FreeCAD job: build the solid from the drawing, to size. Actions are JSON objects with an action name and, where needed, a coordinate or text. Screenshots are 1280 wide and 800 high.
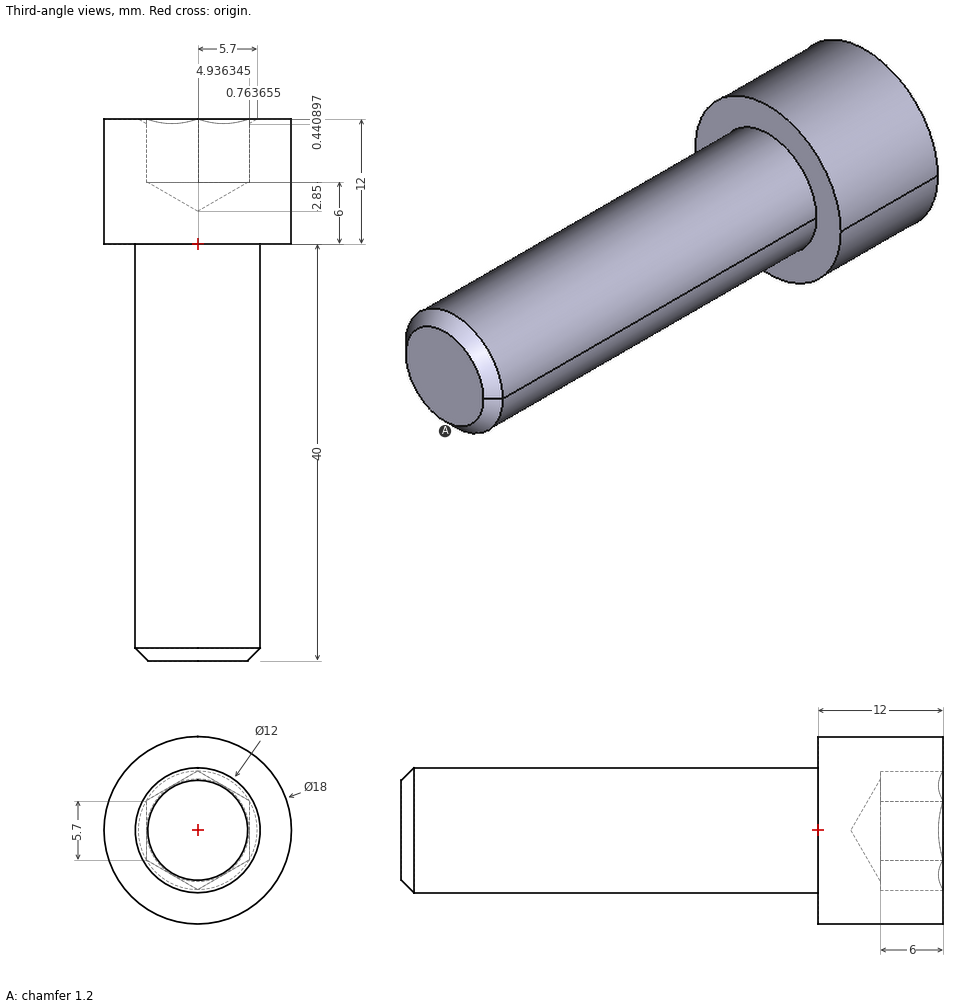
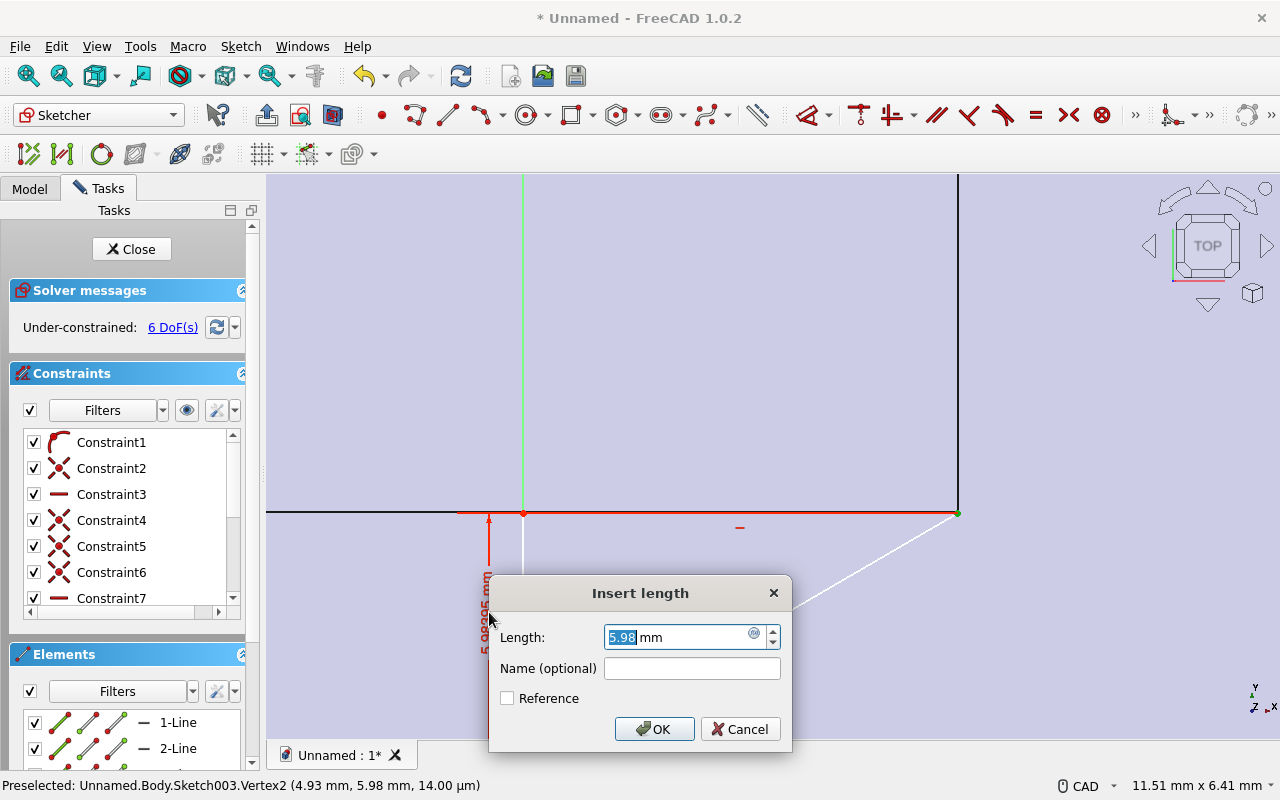
{"action": "type", "text": "6"}
{"action": "key", "text": "Return"}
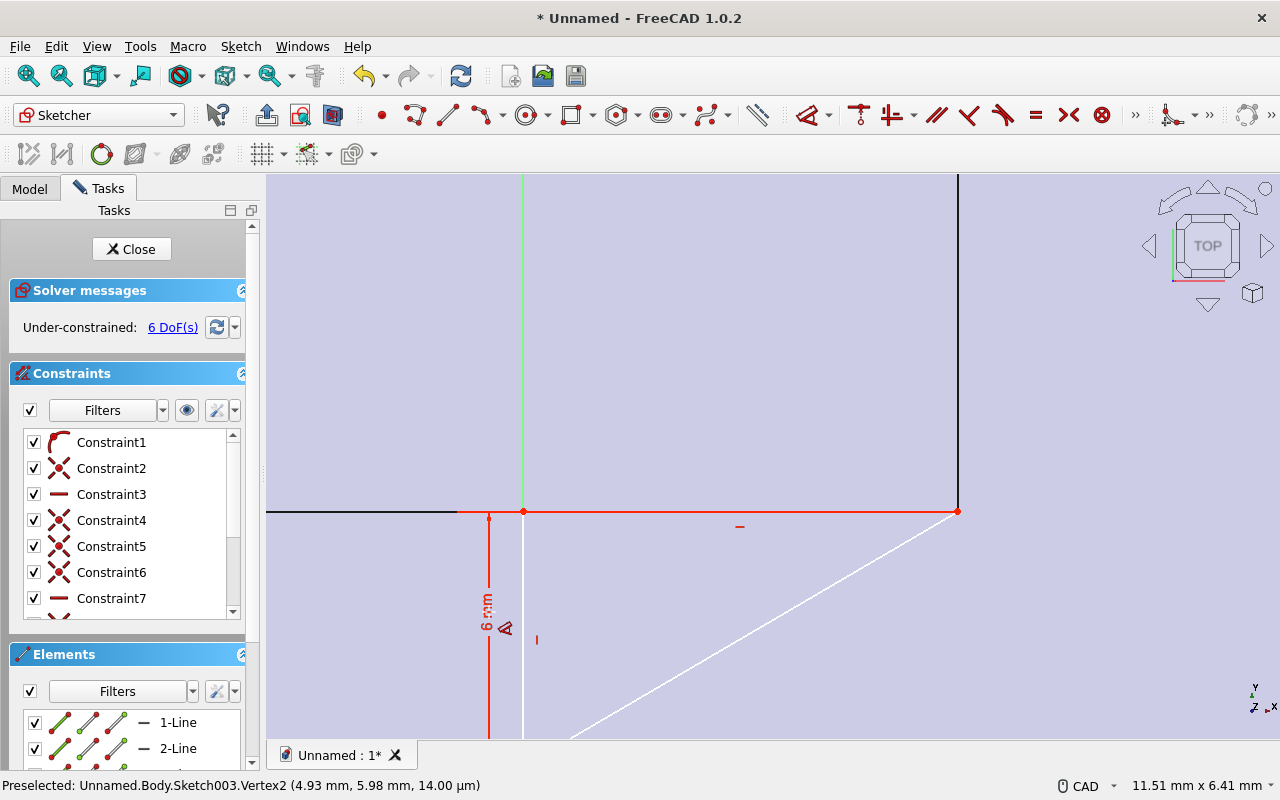
{"action": "scroll", "coordinate": [664, 424], "scroll_direction": "down", "scroll_amount": 5}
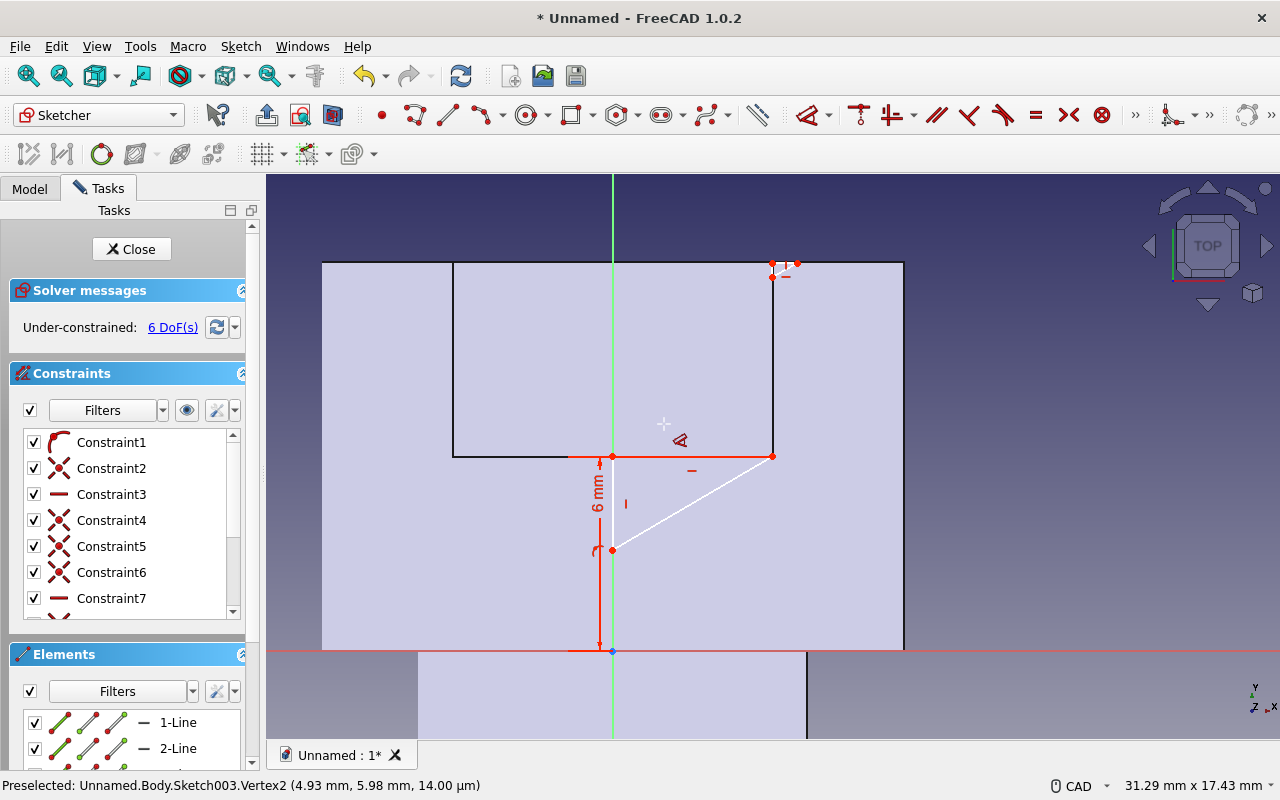
{"action": "left_click", "coordinate": [797, 263]}
{"action": "left_click", "coordinate": [579, 457]}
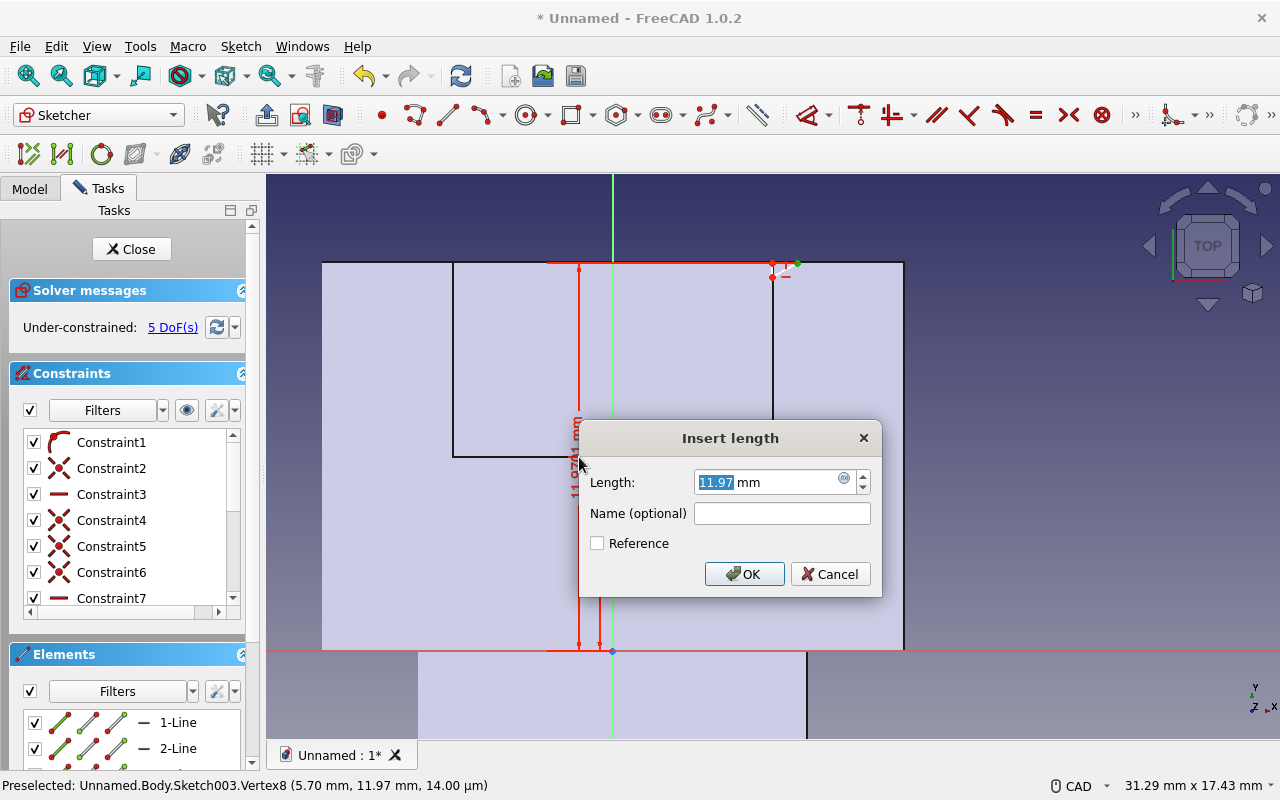
{"action": "type", "text": "12"}
{"action": "key", "text": "Return"}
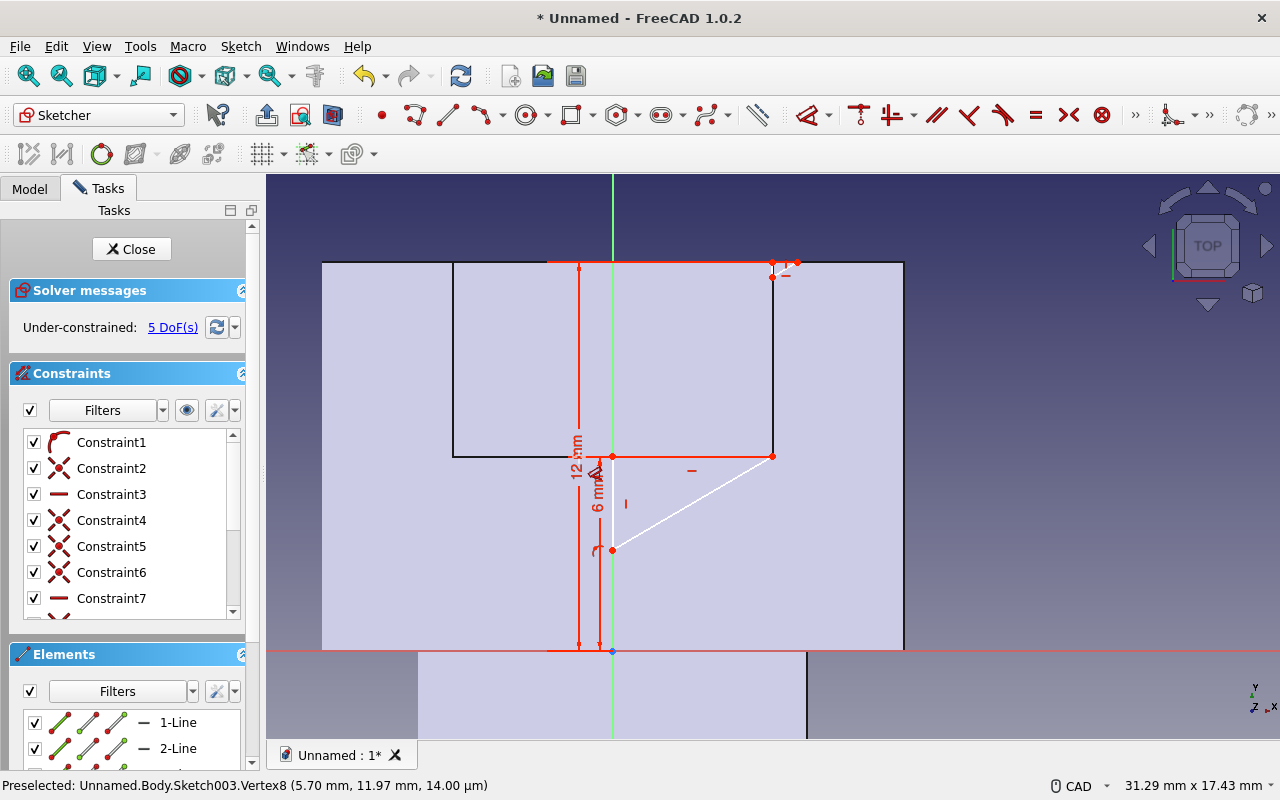
{"action": "left_click", "coordinate": [613, 485]}
{"action": "left_click", "coordinate": [579, 525]}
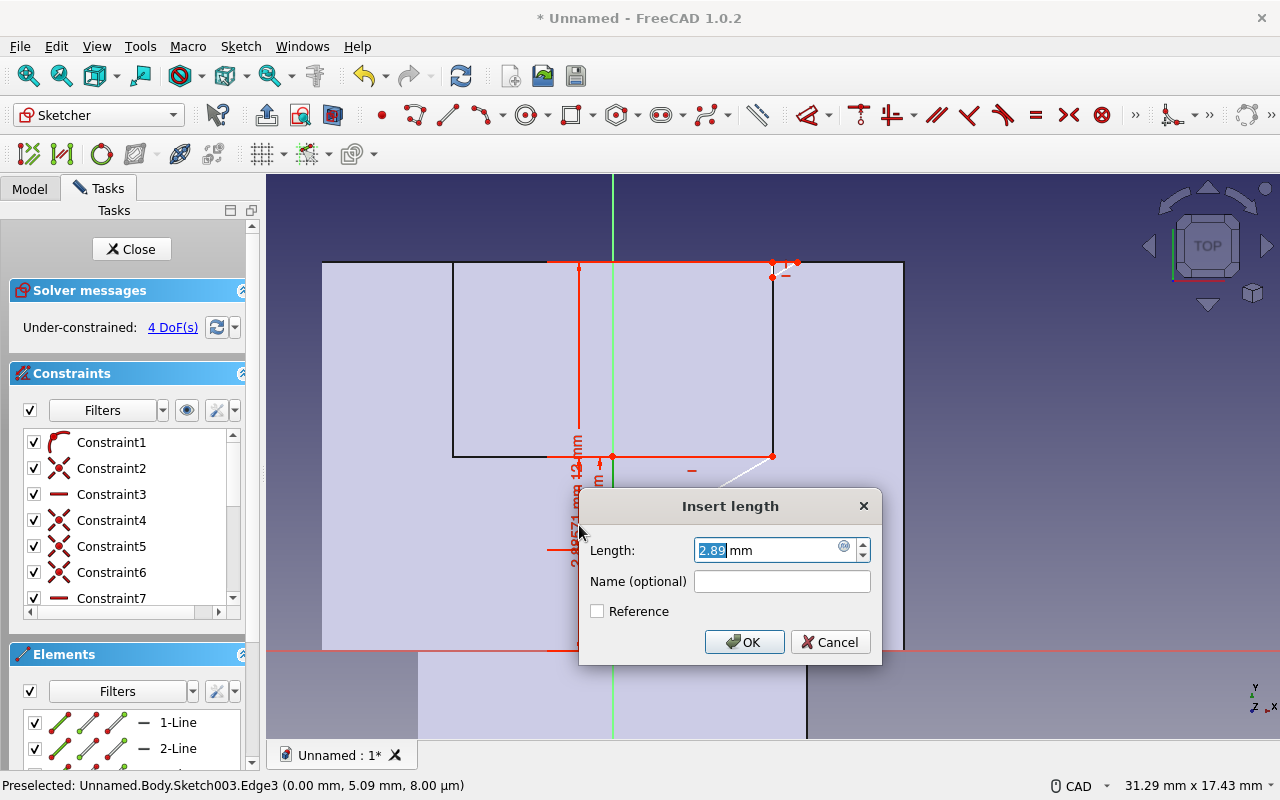
{"action": "type", "text": "2.85"}
{"action": "key", "text": "Return"}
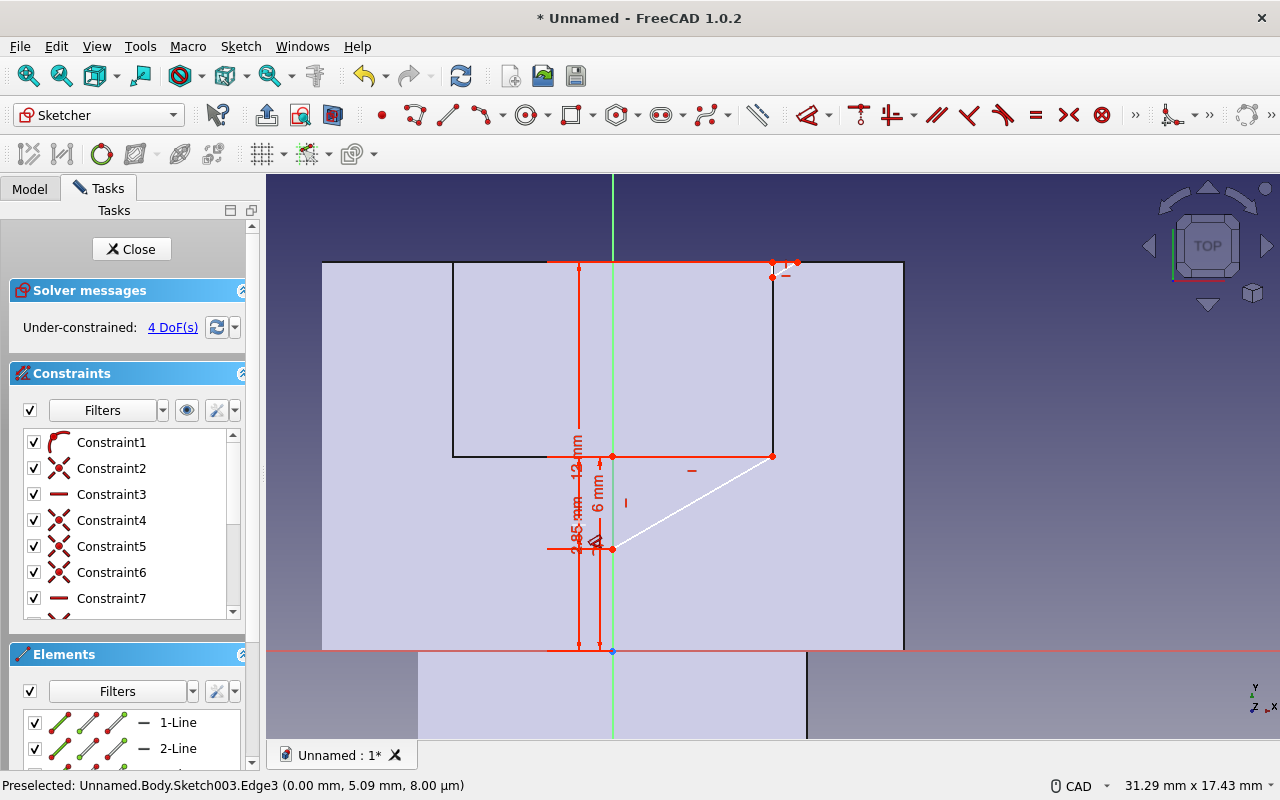
{"action": "left_click", "coordinate": [797, 262]}
{"action": "left_click", "coordinate": [705, 685]}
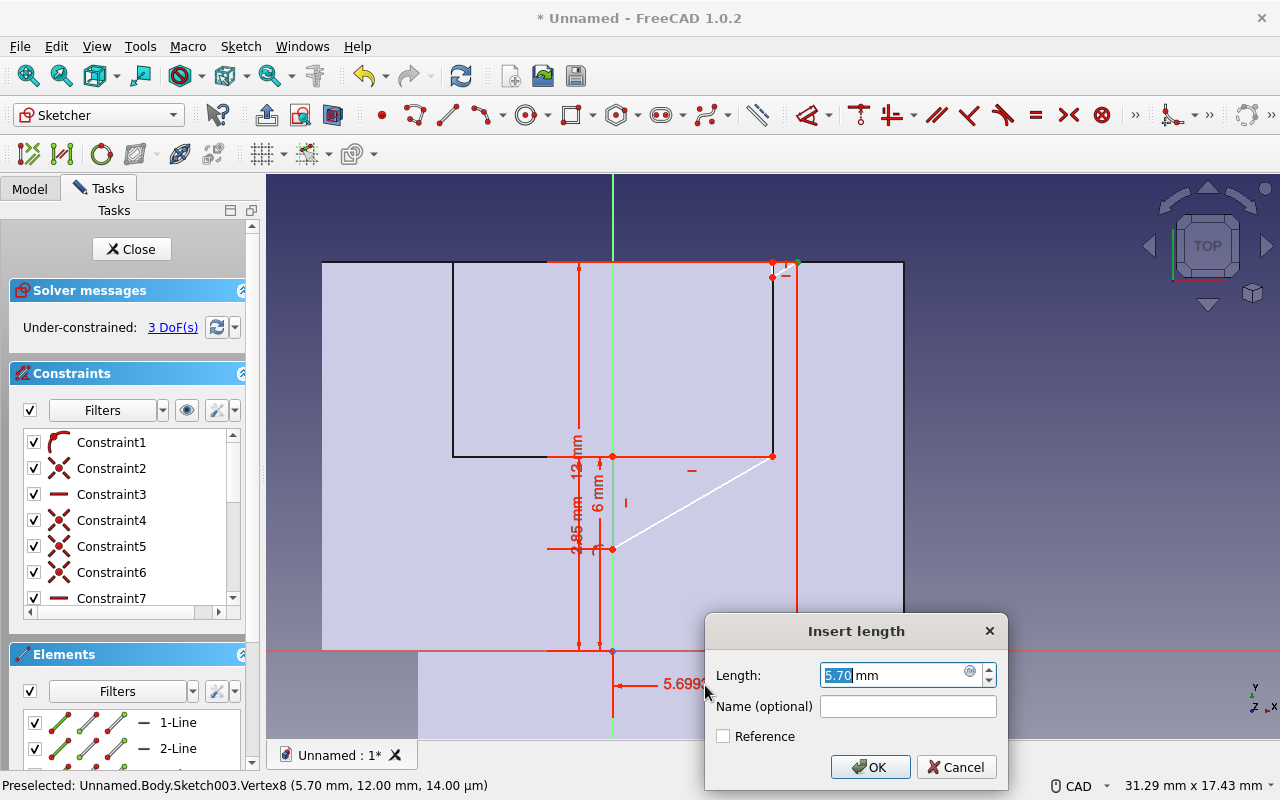
{"action": "type", "text": "5.7"}
{"action": "key", "text": "Return"}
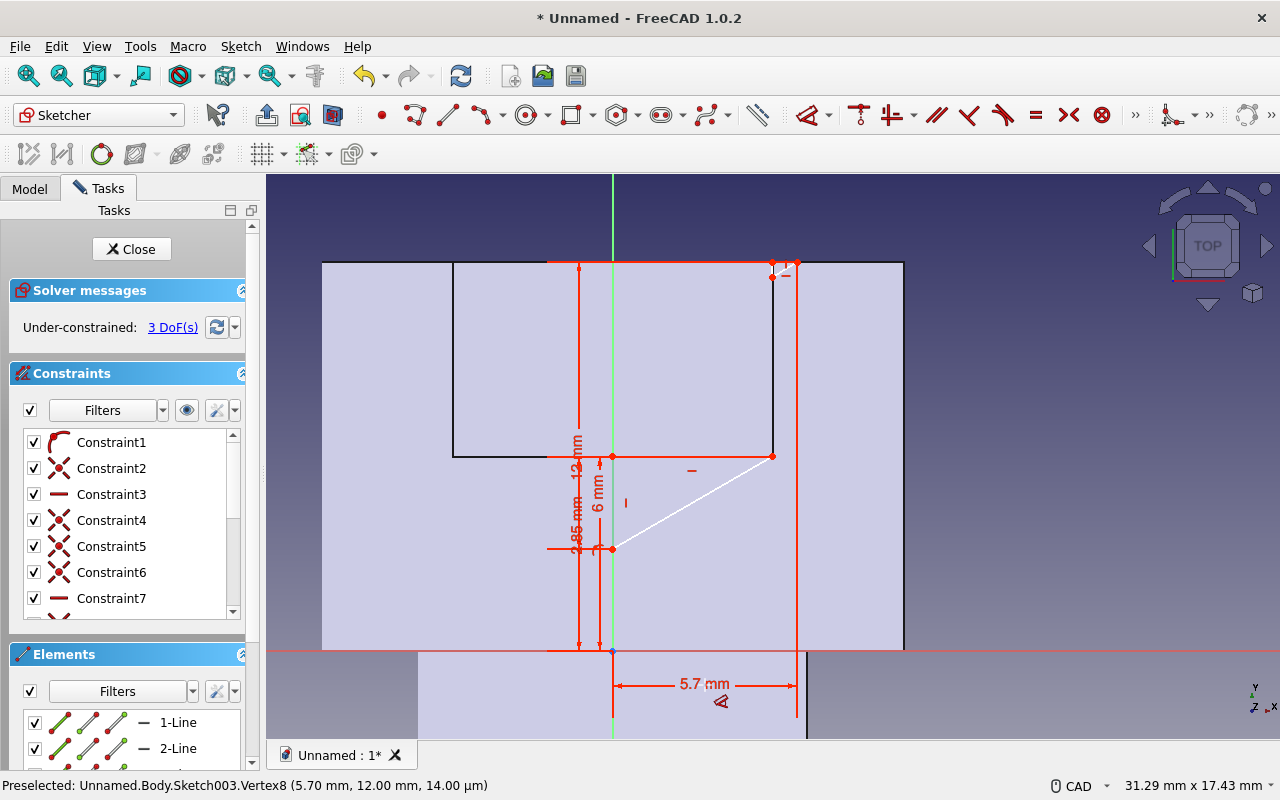
{"action": "left_click", "coordinate": [724, 457]}
{"action": "left_click", "coordinate": [748, 491]}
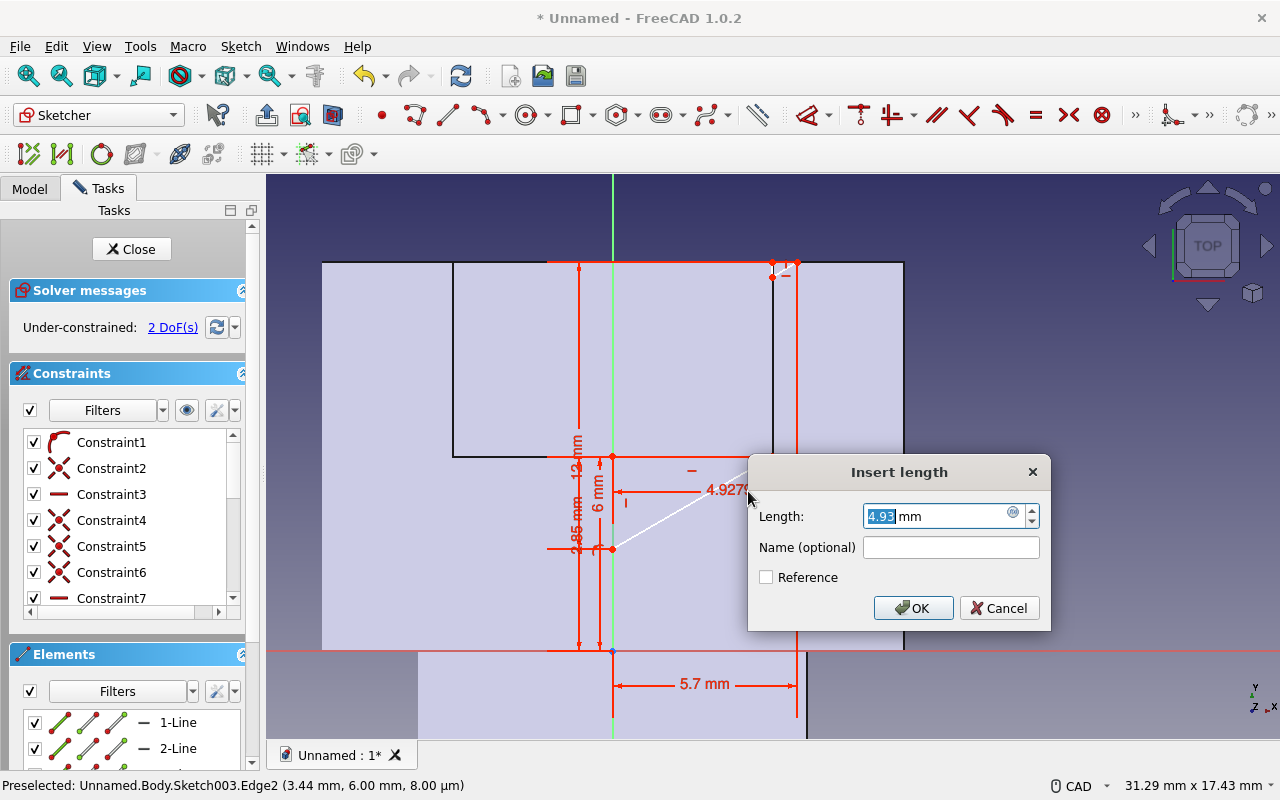
{"action": "type", "text": "4.936345"}
{"action": "key", "text": "Return"}